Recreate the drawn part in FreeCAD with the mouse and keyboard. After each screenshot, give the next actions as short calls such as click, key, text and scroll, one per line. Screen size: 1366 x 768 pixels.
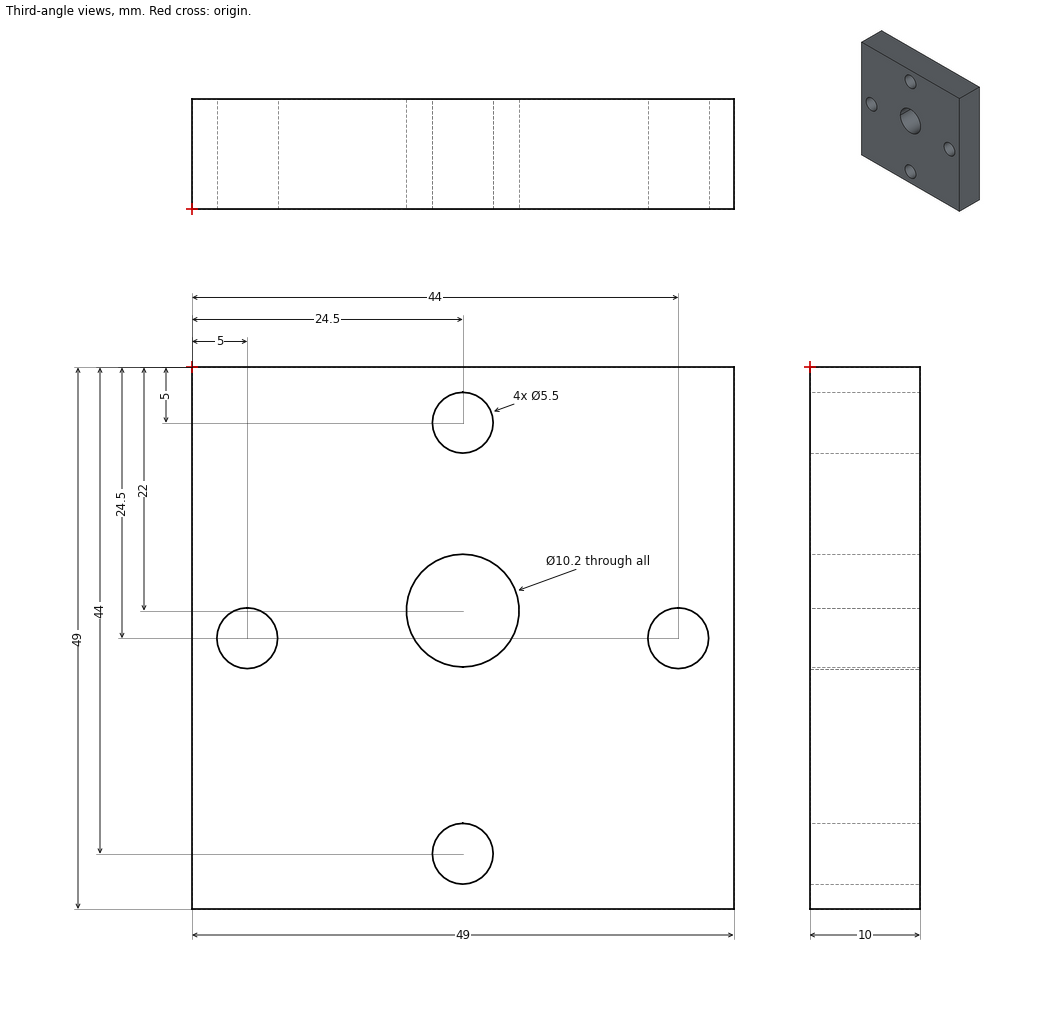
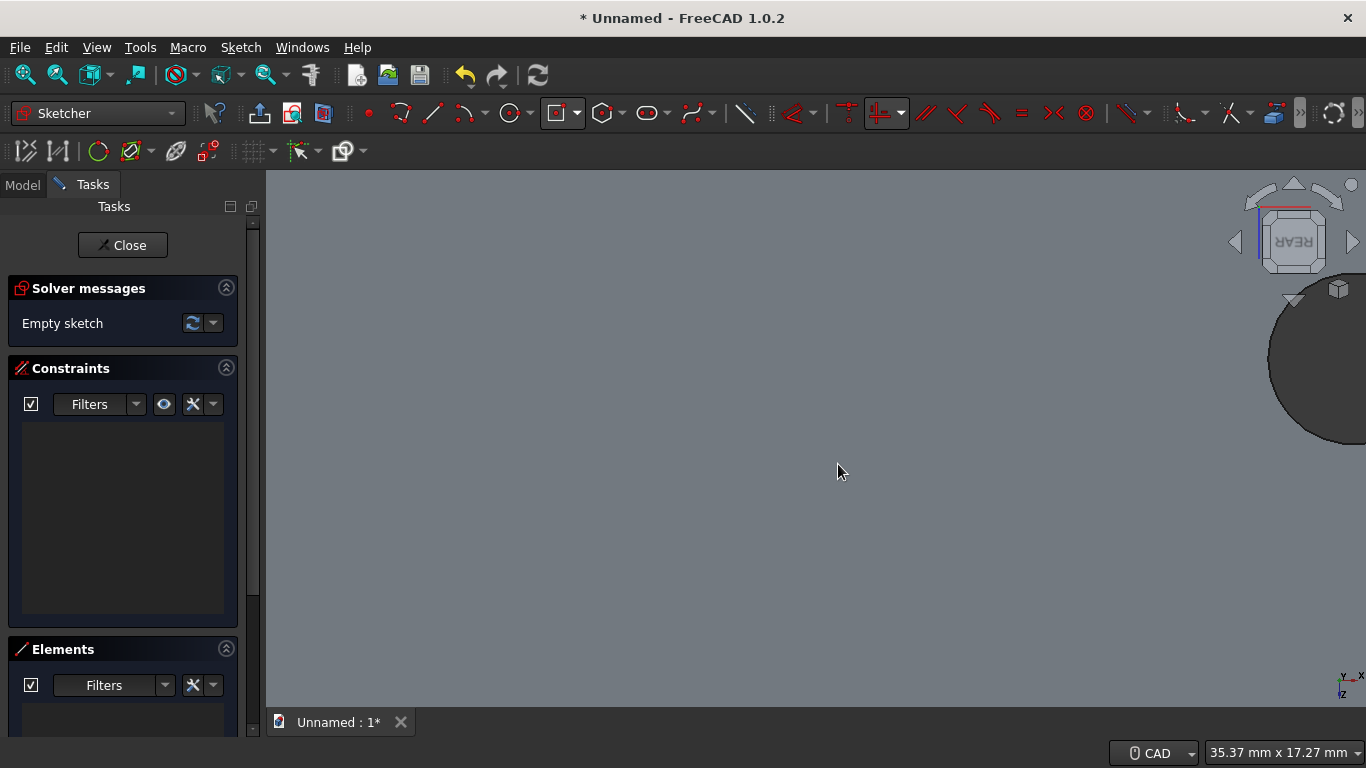
click(510, 114)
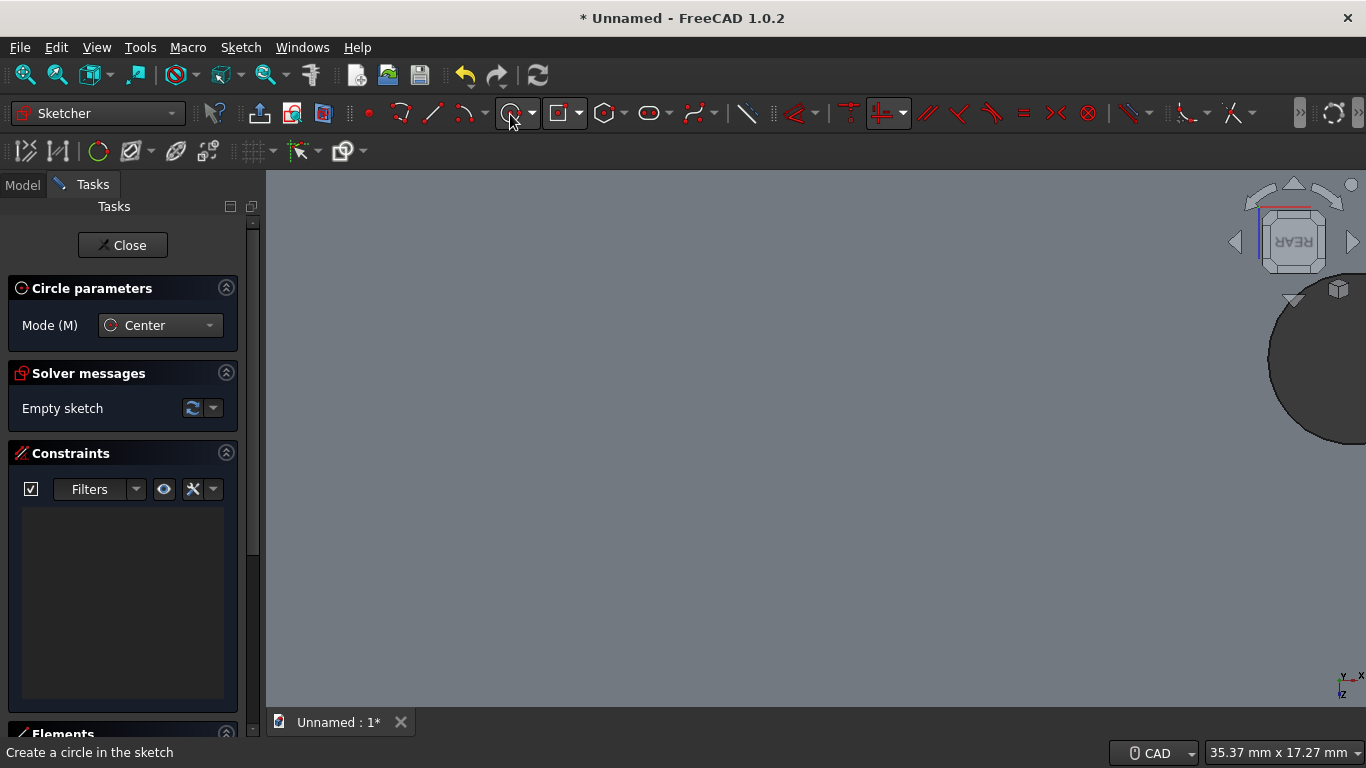
click(747, 437)
click(859, 325)
key(Escape)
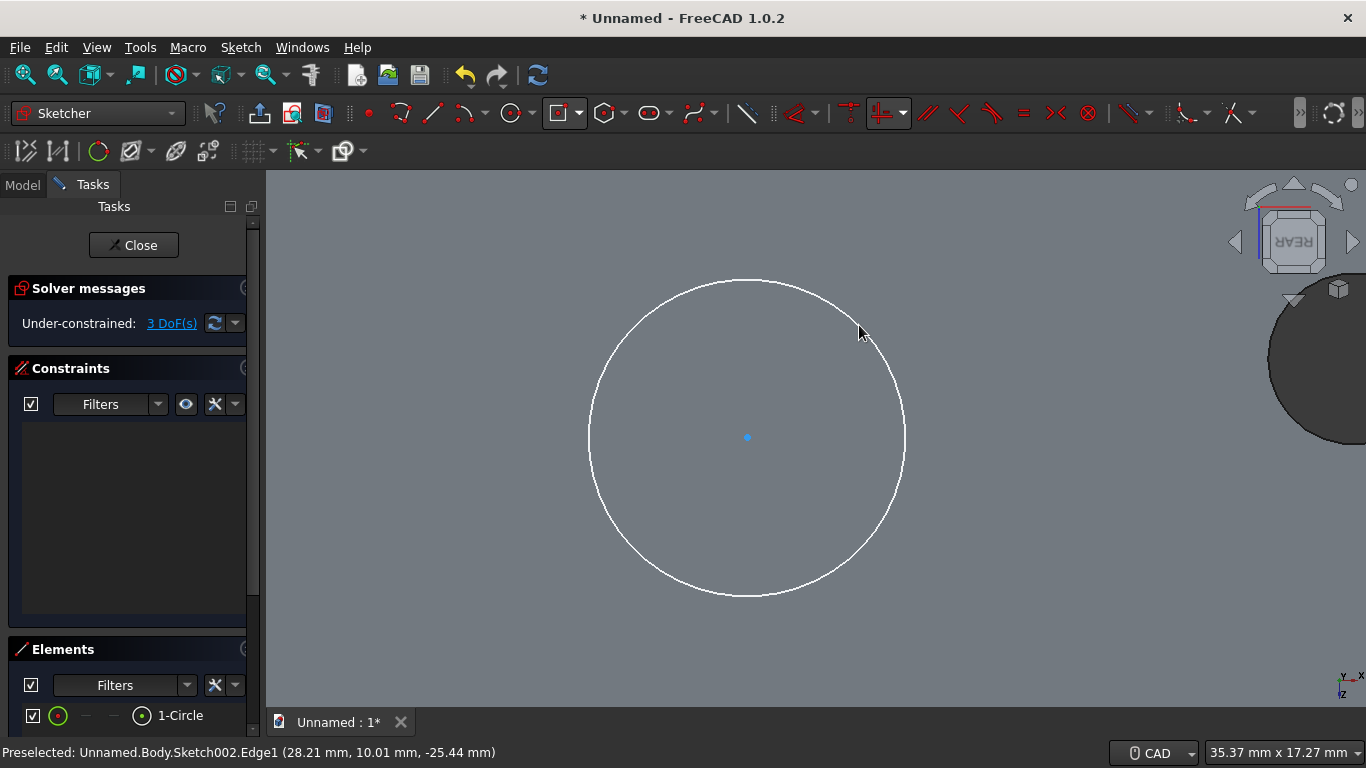
click(794, 114)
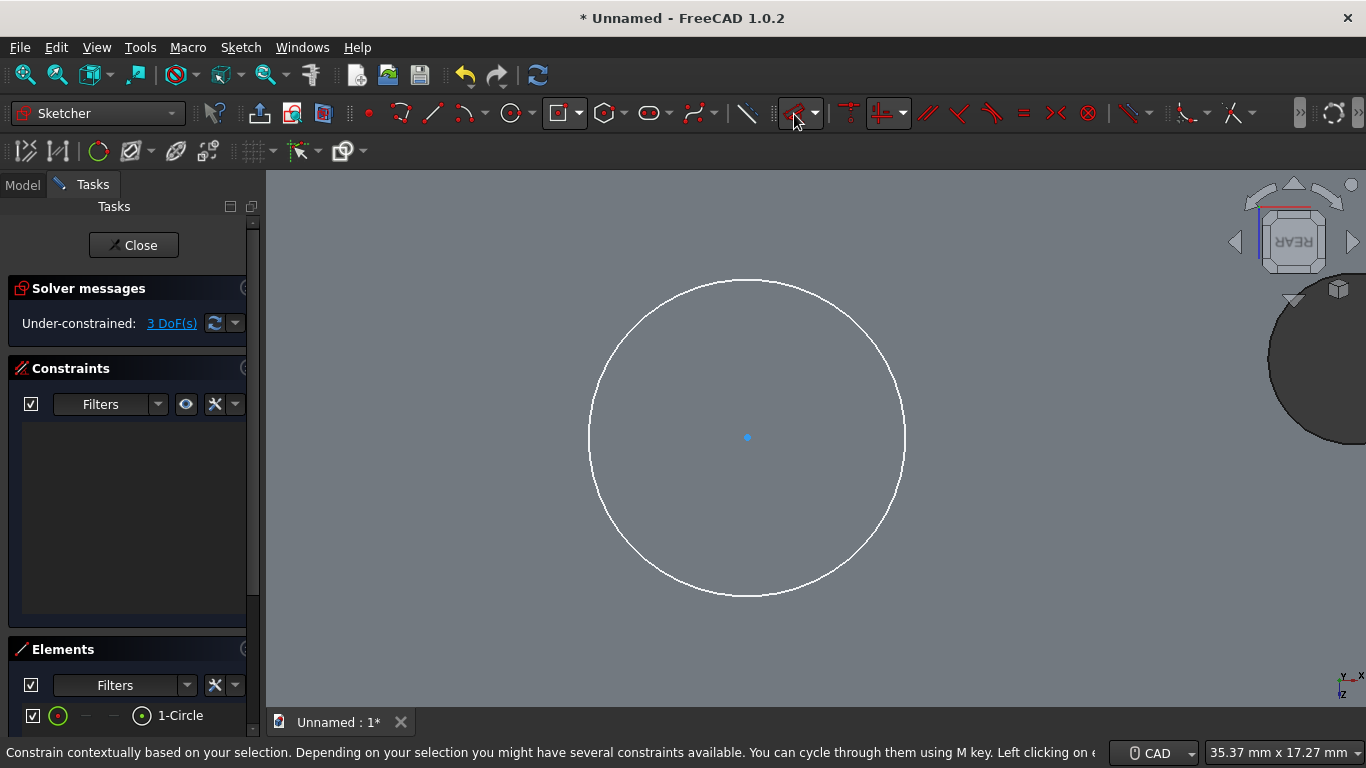
click(859, 326)
click(882, 303)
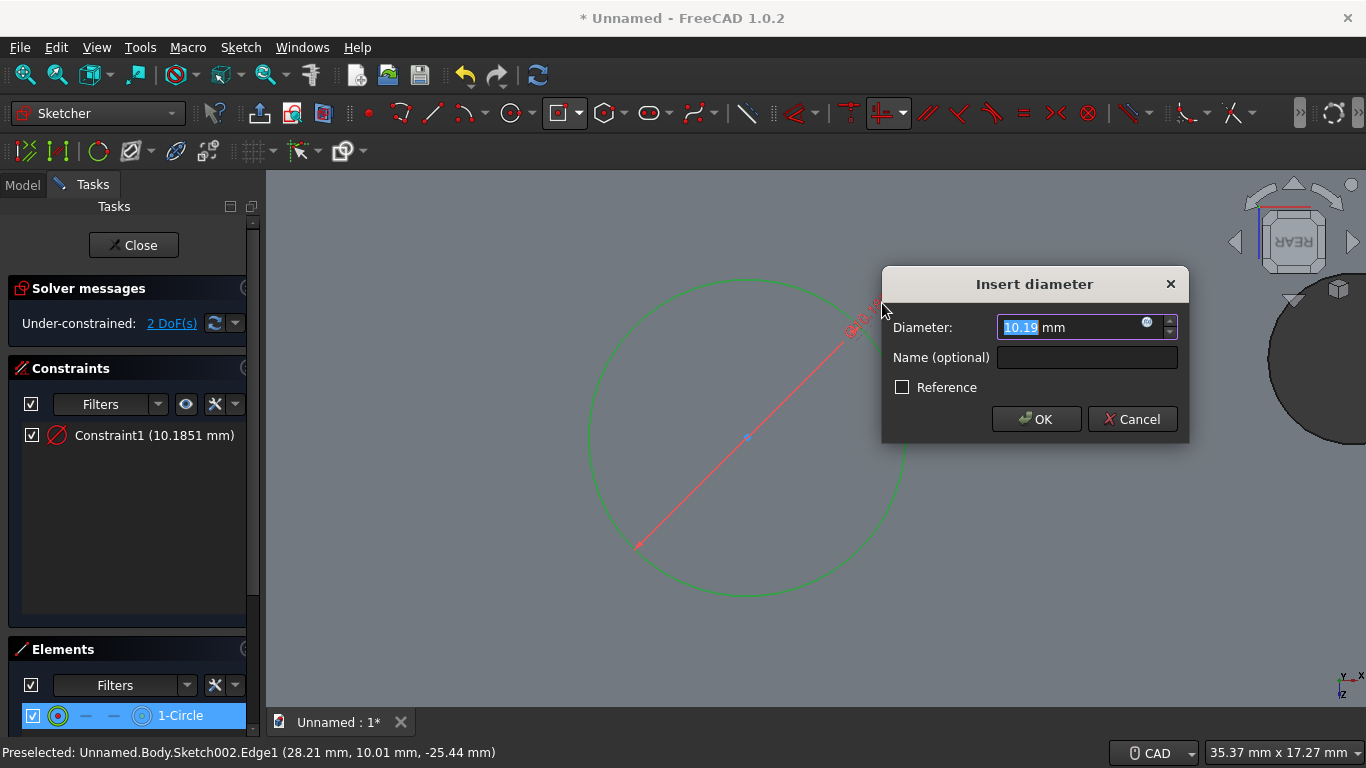
text(10.2)
key(Return)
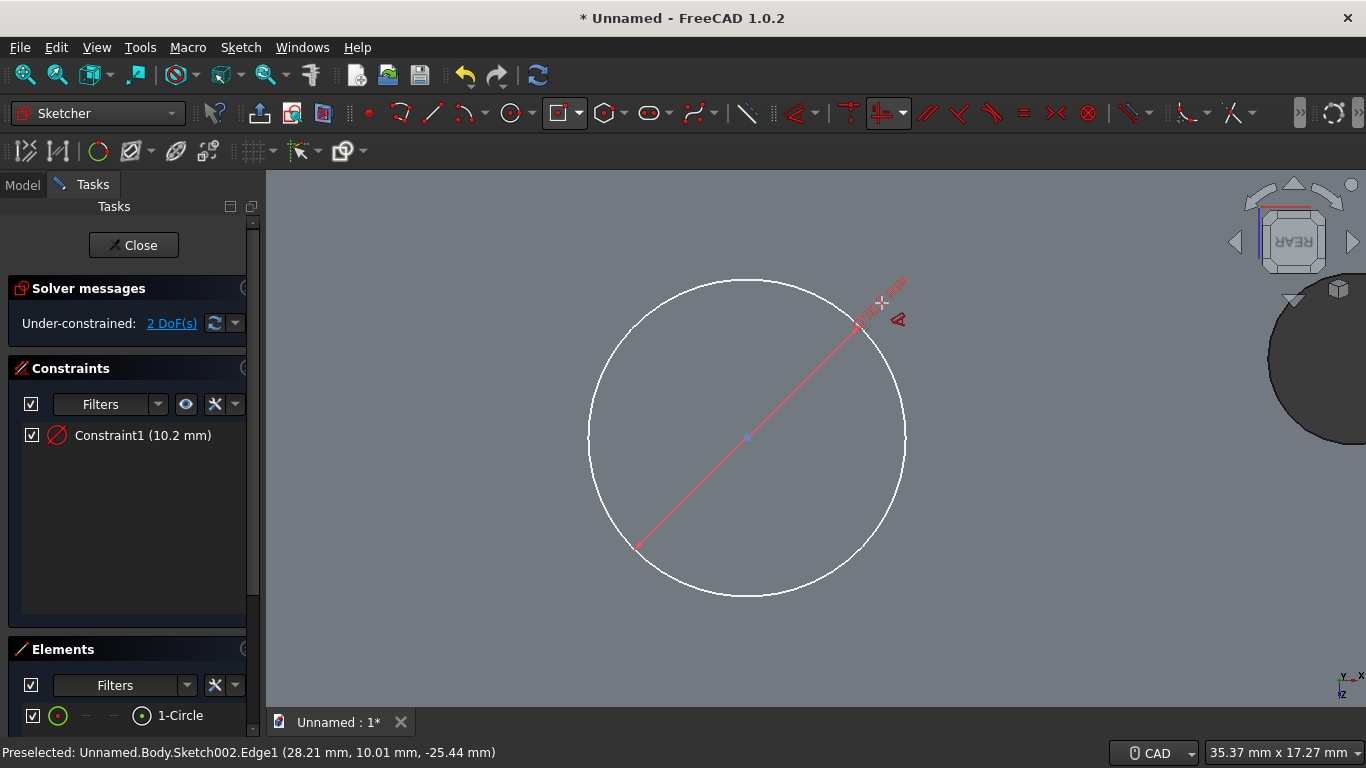
click(747, 438)
click(781, 559)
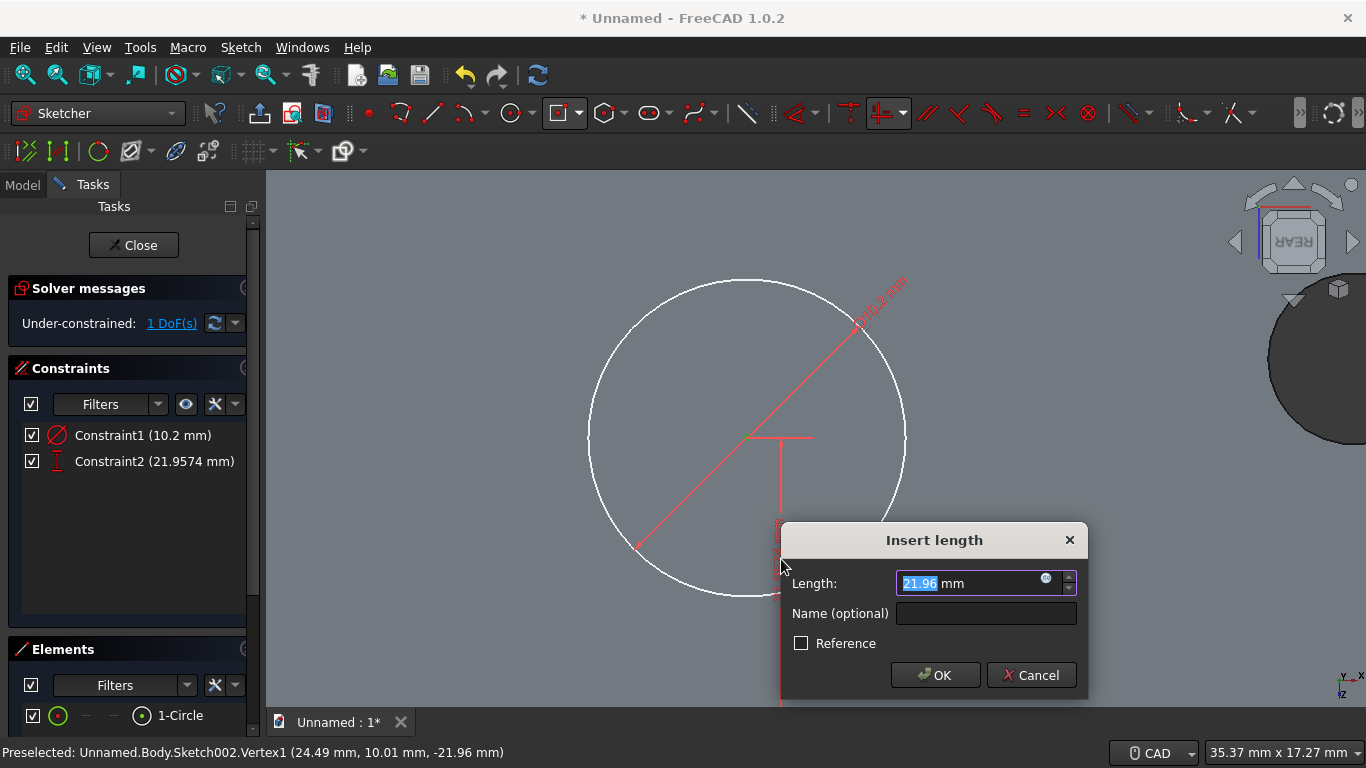
text(22)
key(Return)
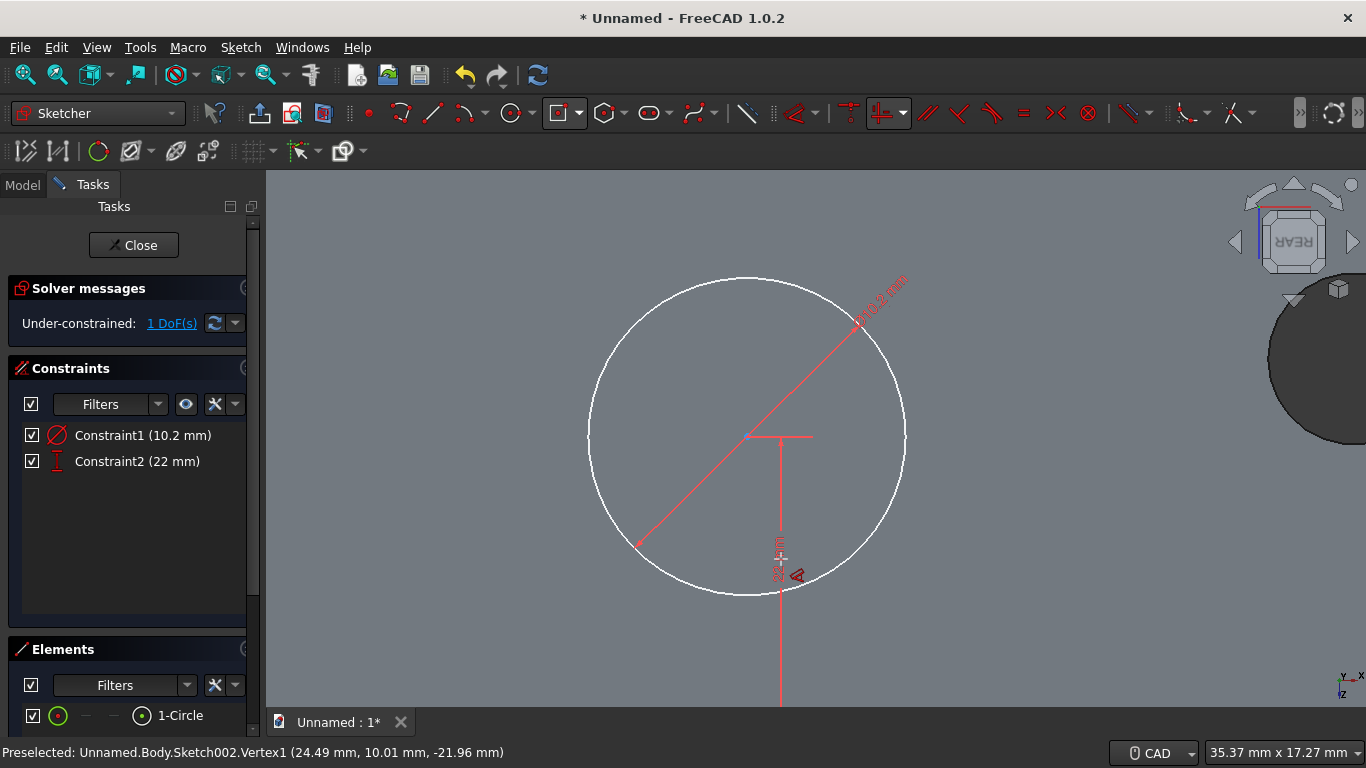
click(747, 437)
click(520, 403)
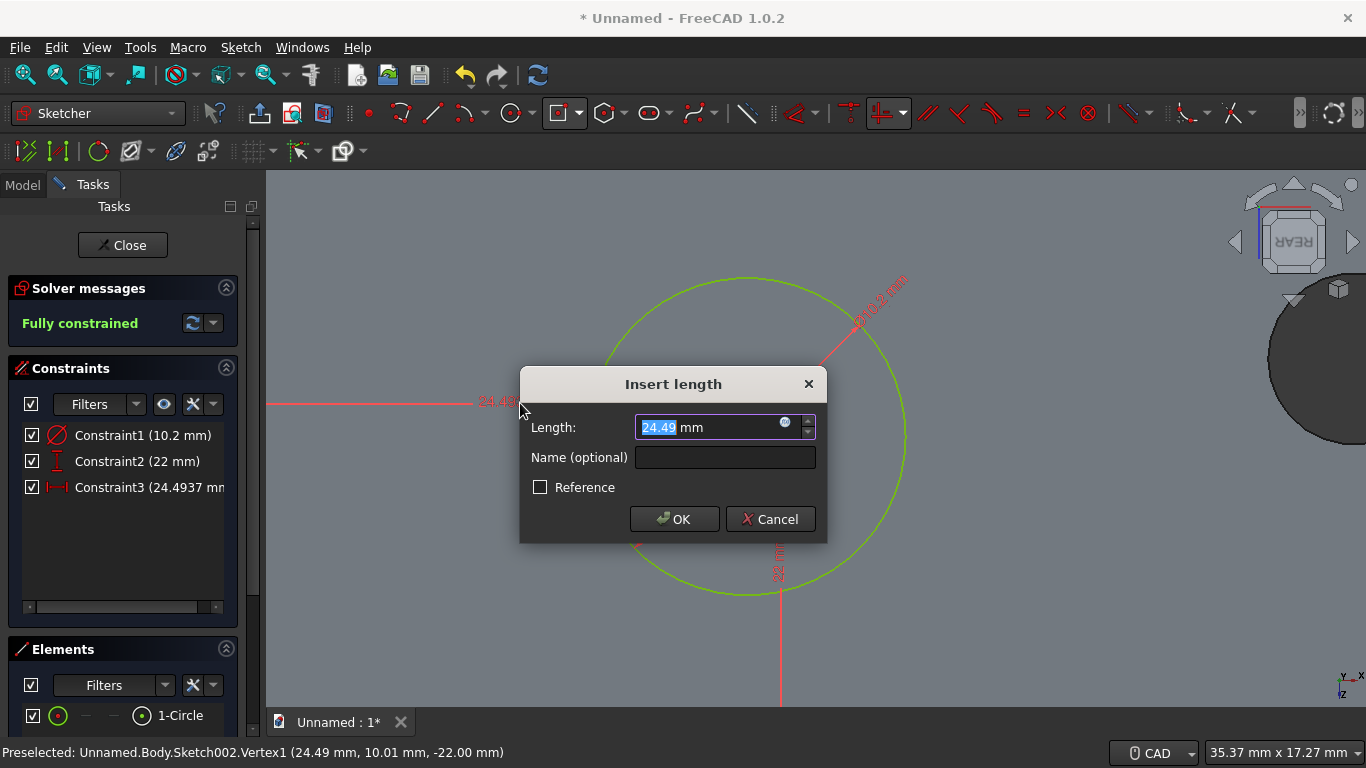
text(24.5)
key(Return)
key(Escape)